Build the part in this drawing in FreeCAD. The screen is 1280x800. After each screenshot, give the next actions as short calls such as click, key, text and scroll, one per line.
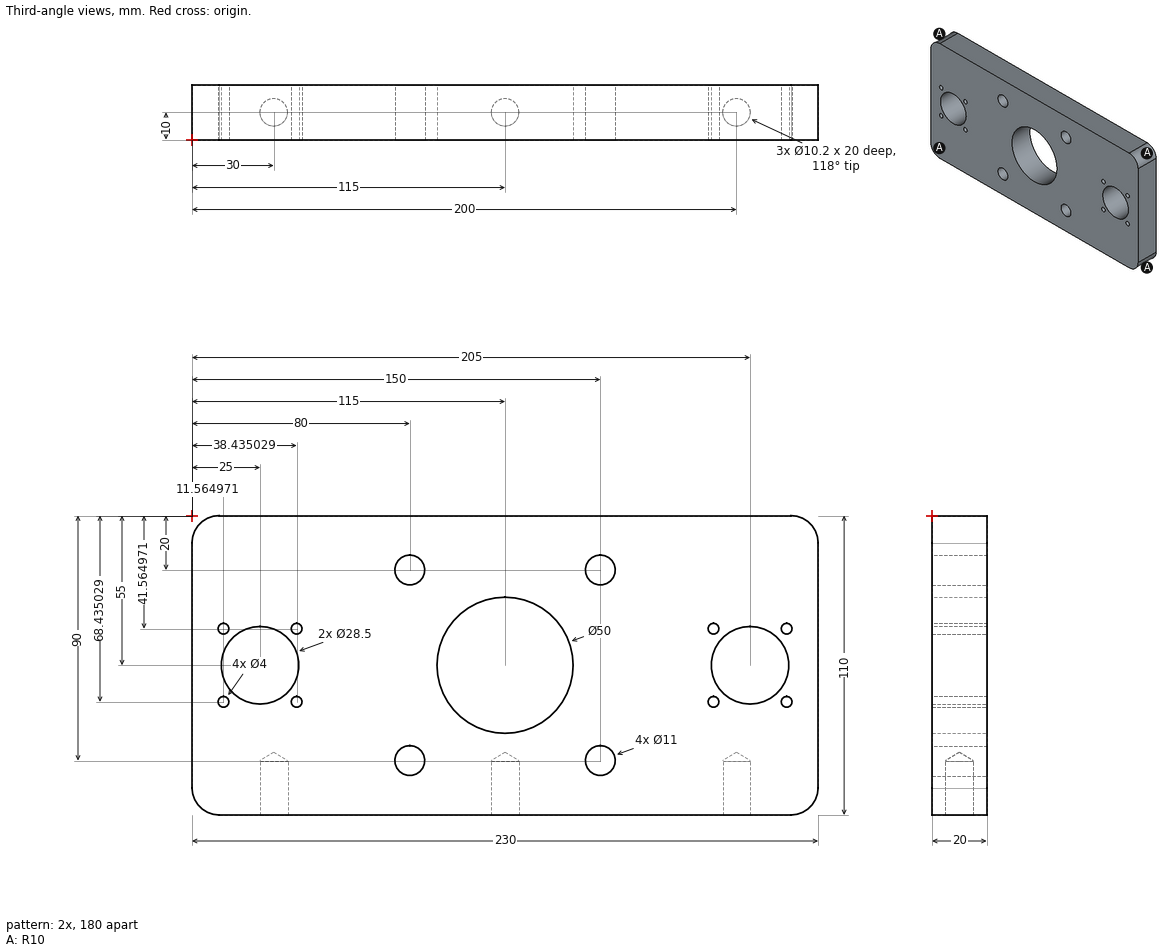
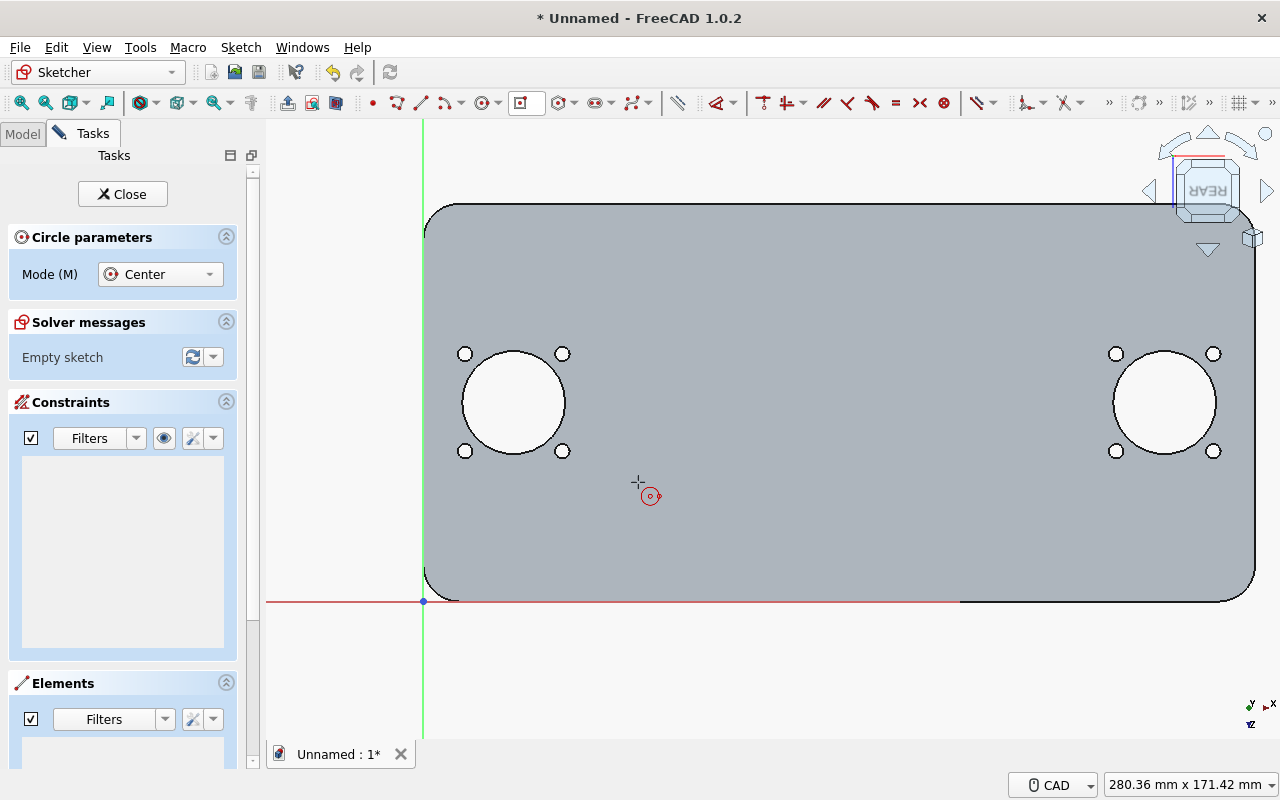
click(839, 403)
move(903, 339)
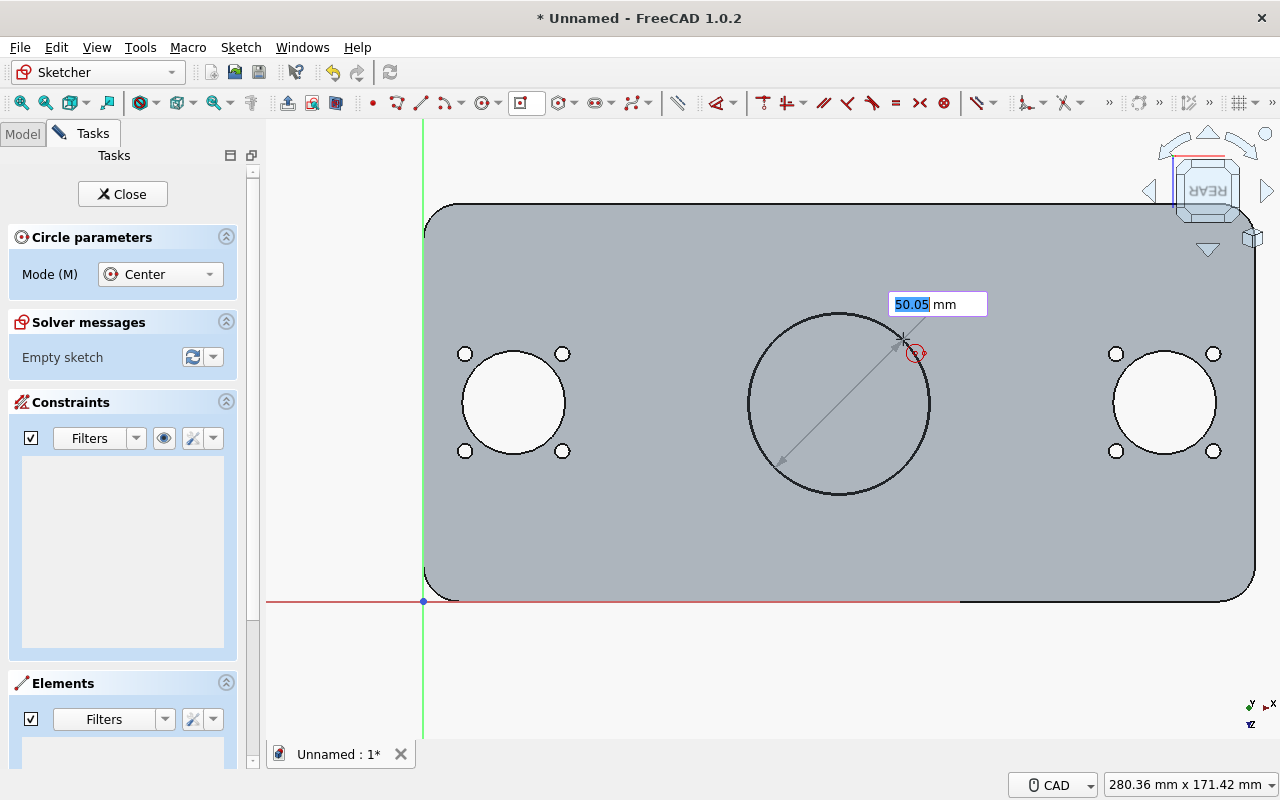
text(50)
key(Return)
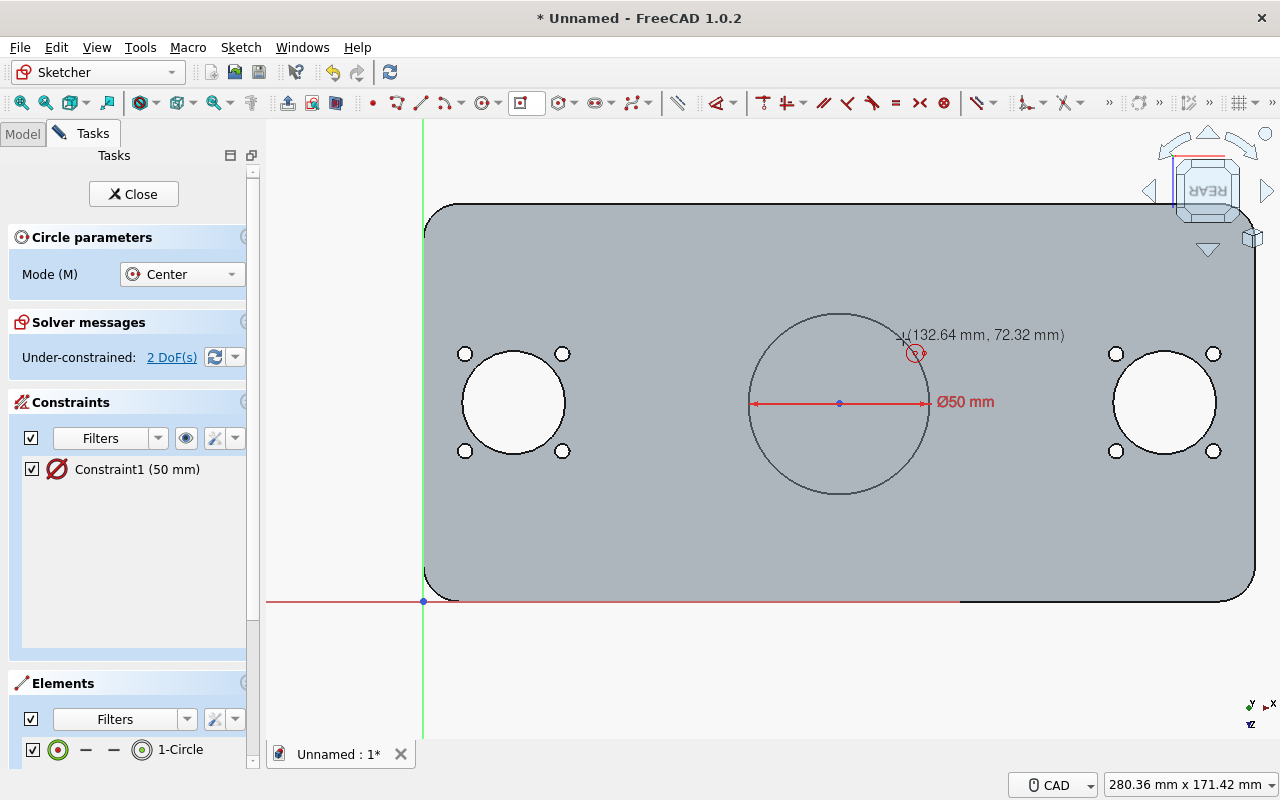
click(966, 276)
move(980, 262)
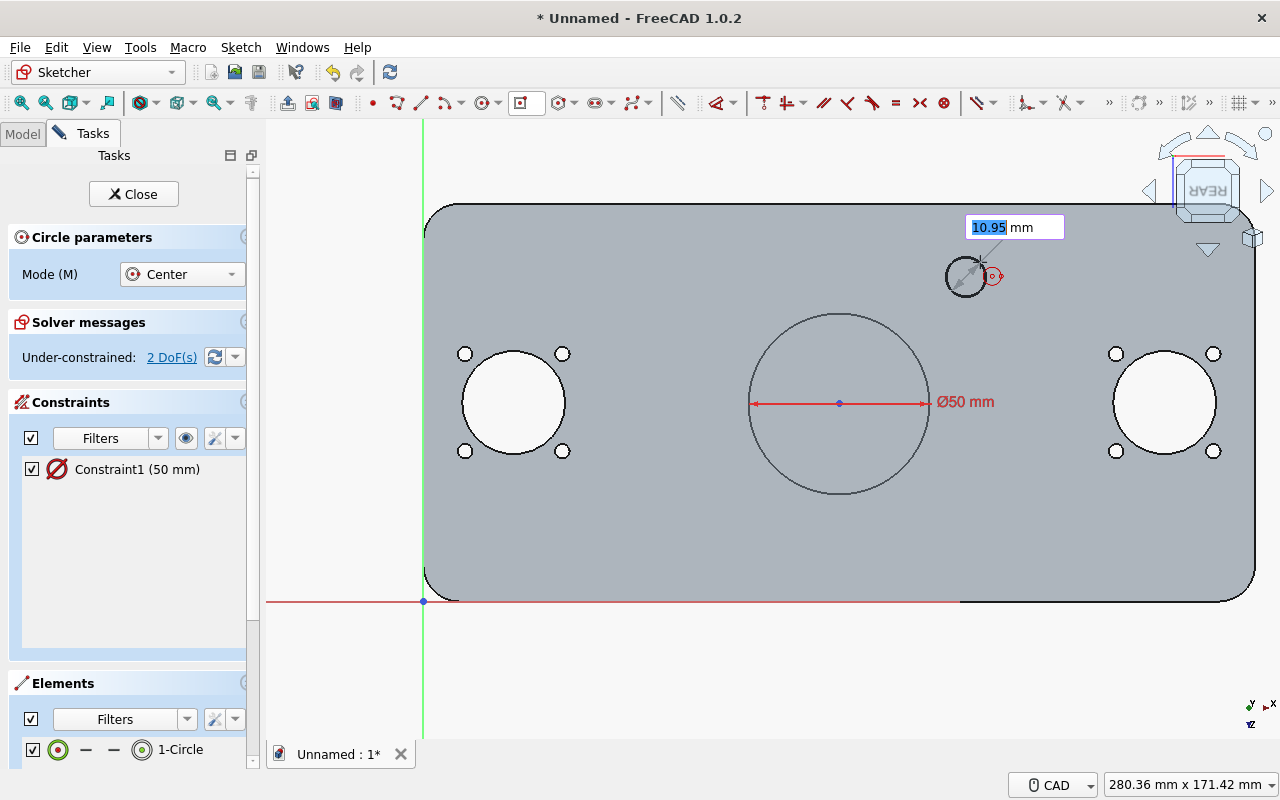
text(11)
key(Return)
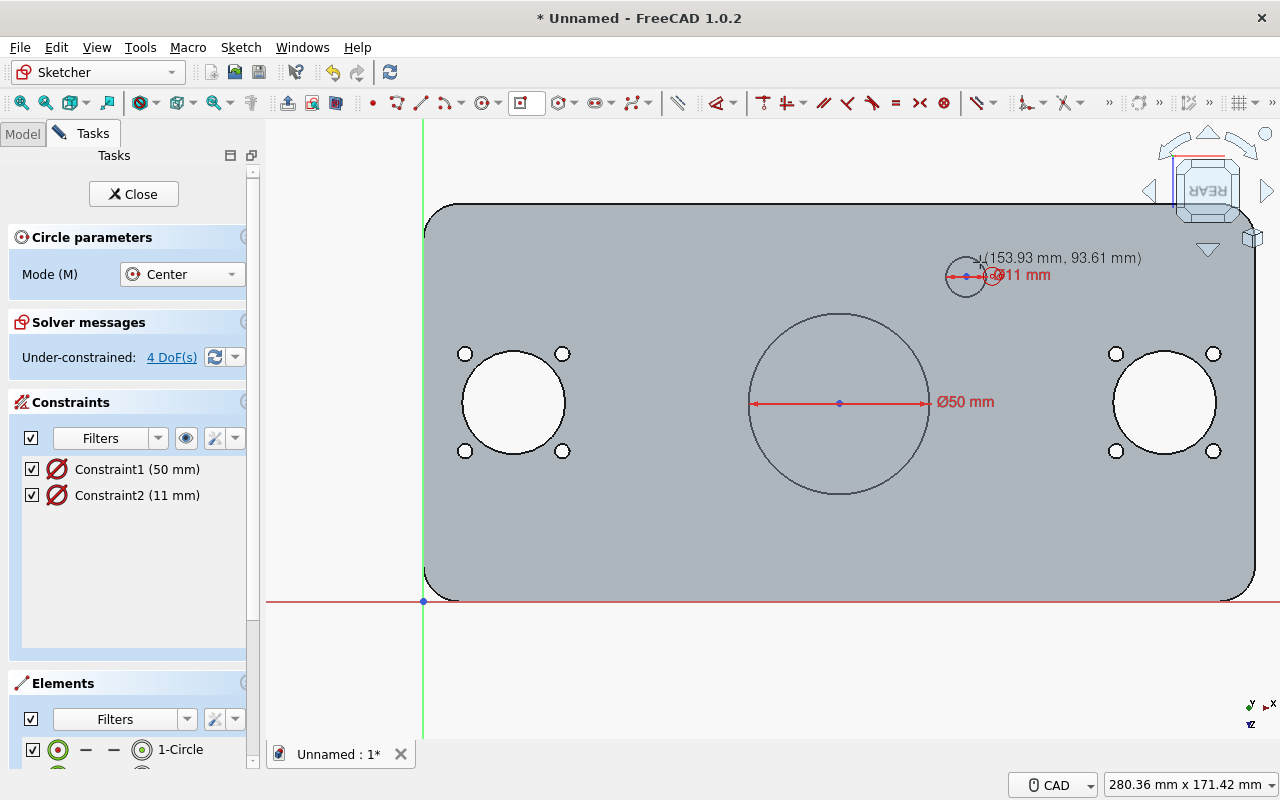
click(966, 529)
move(980, 515)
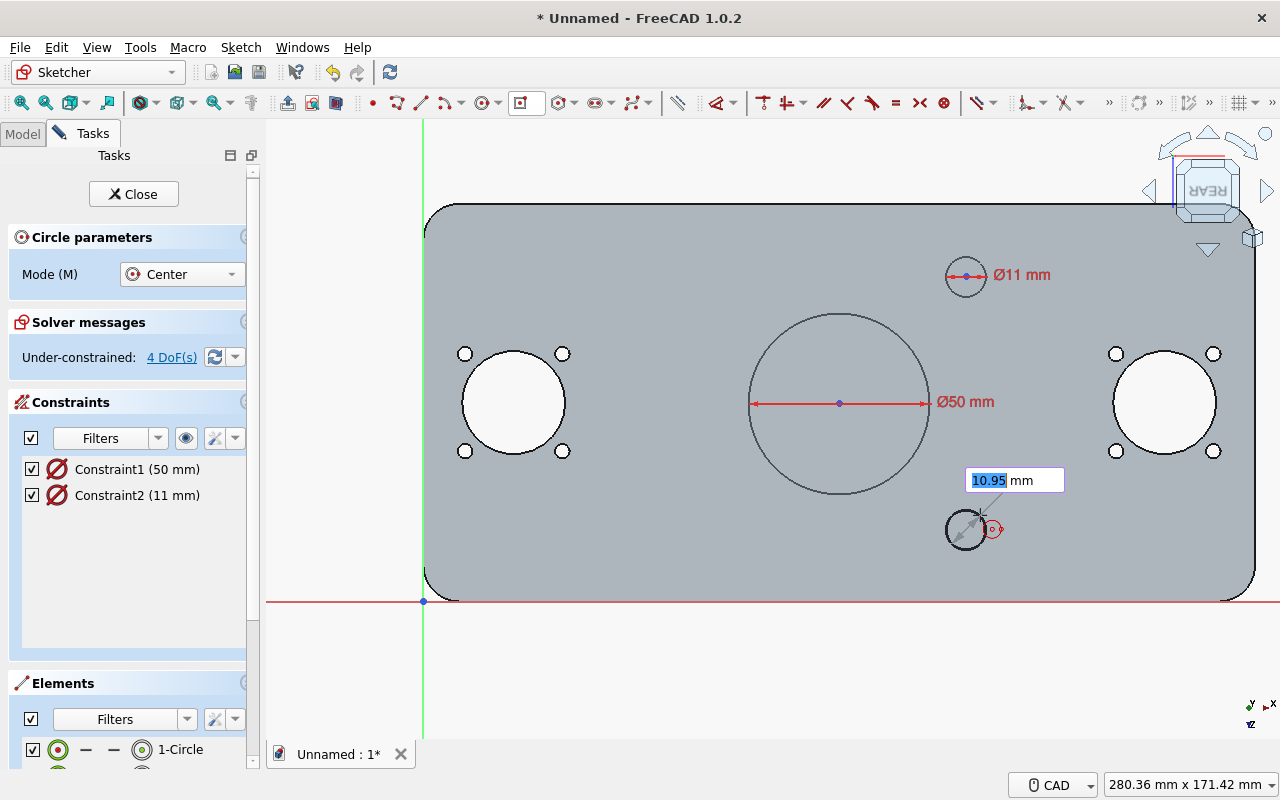
text(11)
key(Return)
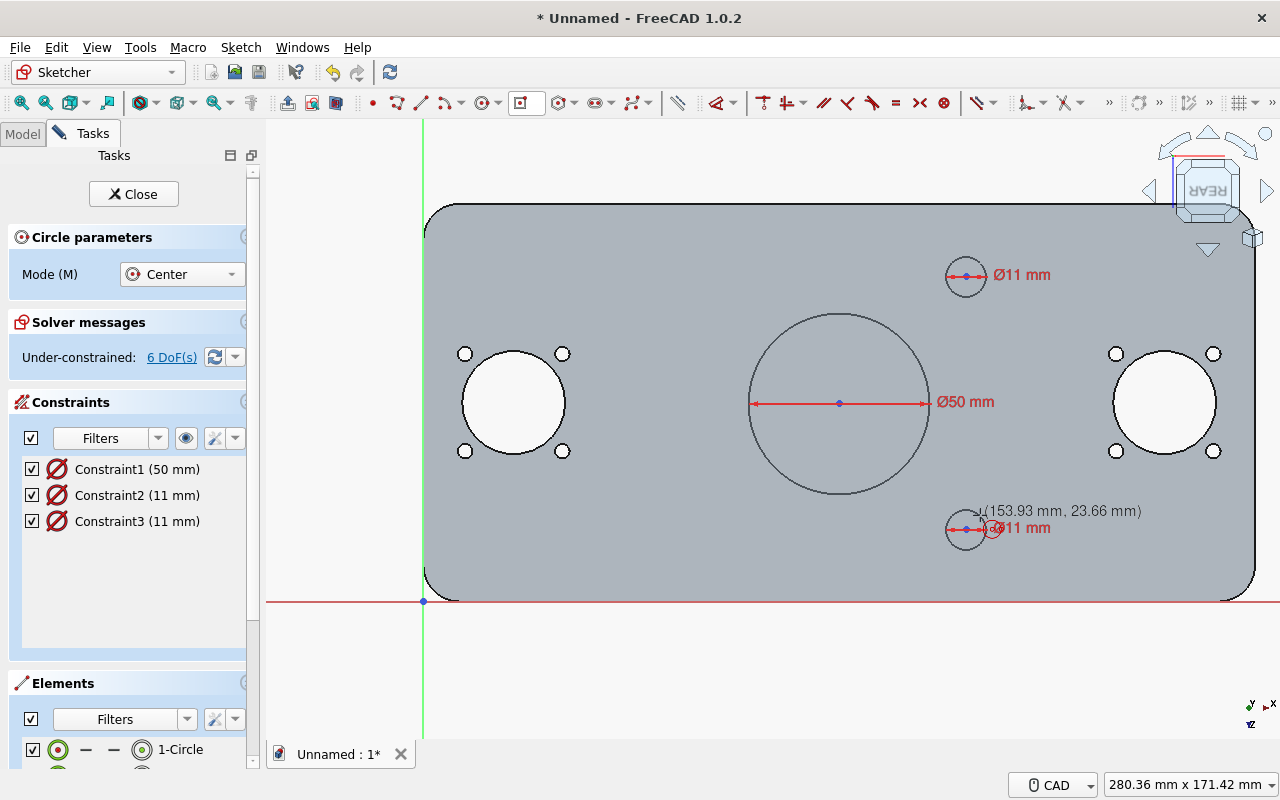
click(713, 529)
move(727, 515)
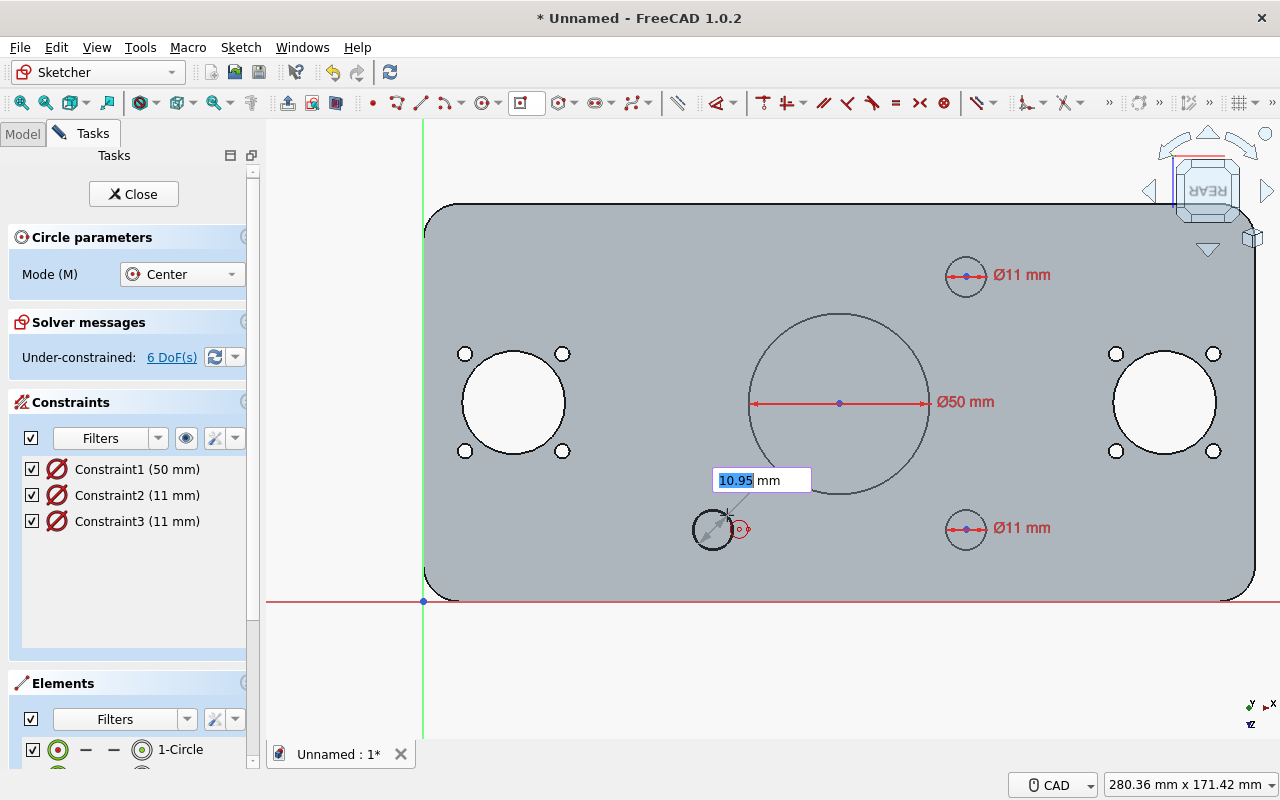
text(11)
key(Return)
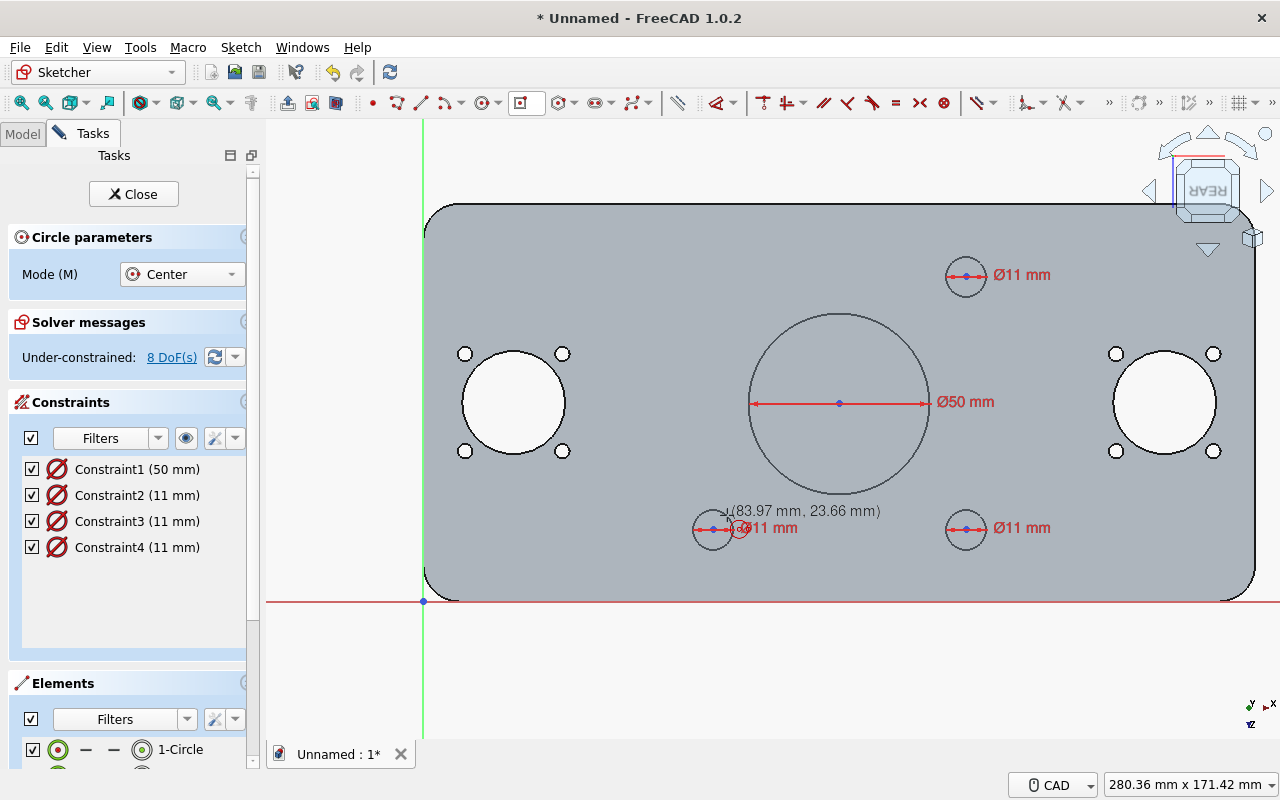
click(713, 276)
move(727, 262)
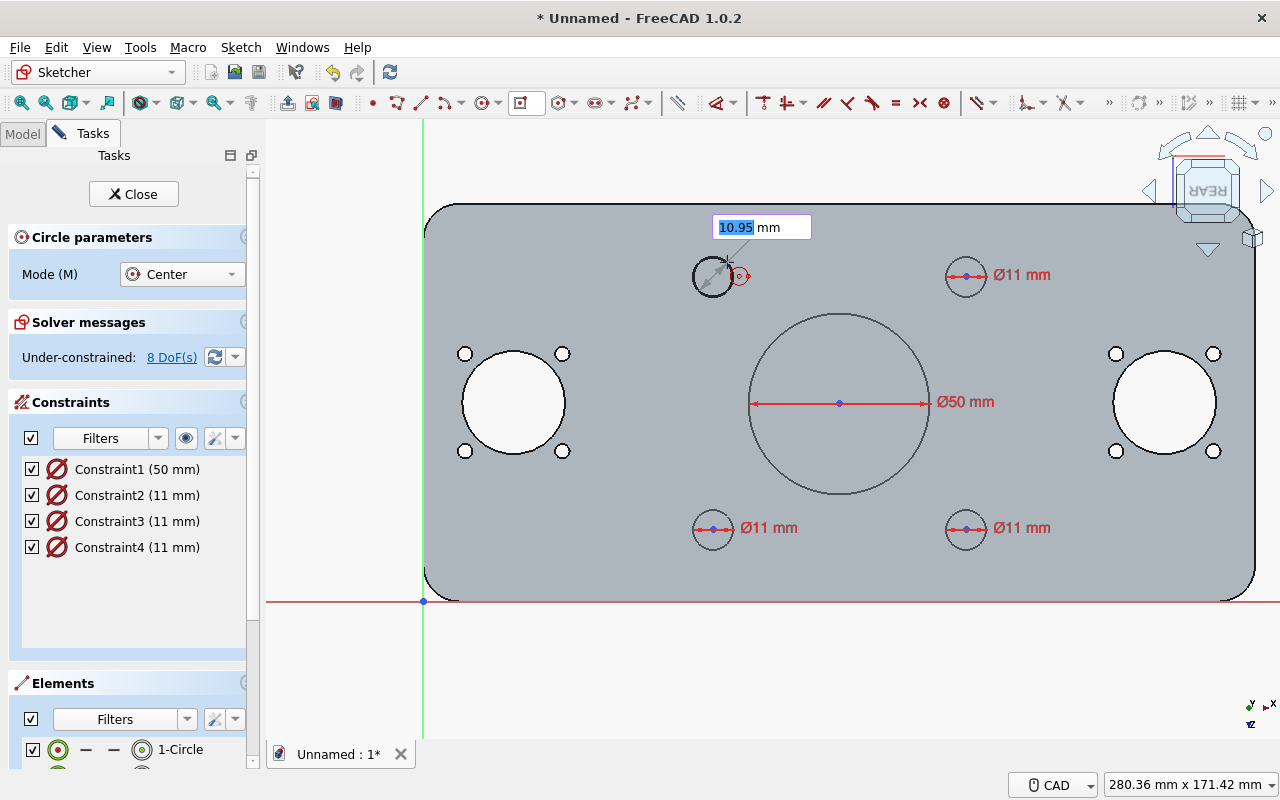
text(11)
key(Return)
key(Escape)